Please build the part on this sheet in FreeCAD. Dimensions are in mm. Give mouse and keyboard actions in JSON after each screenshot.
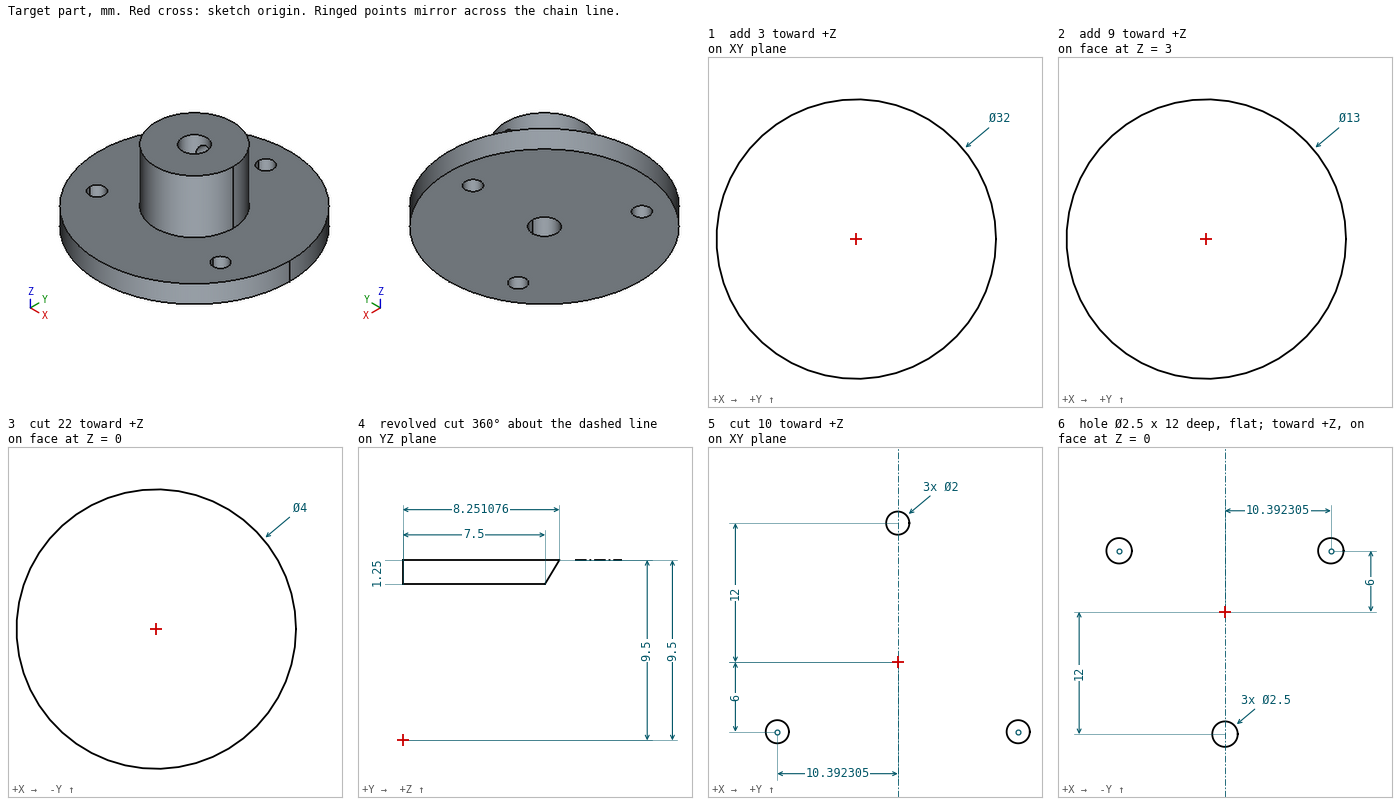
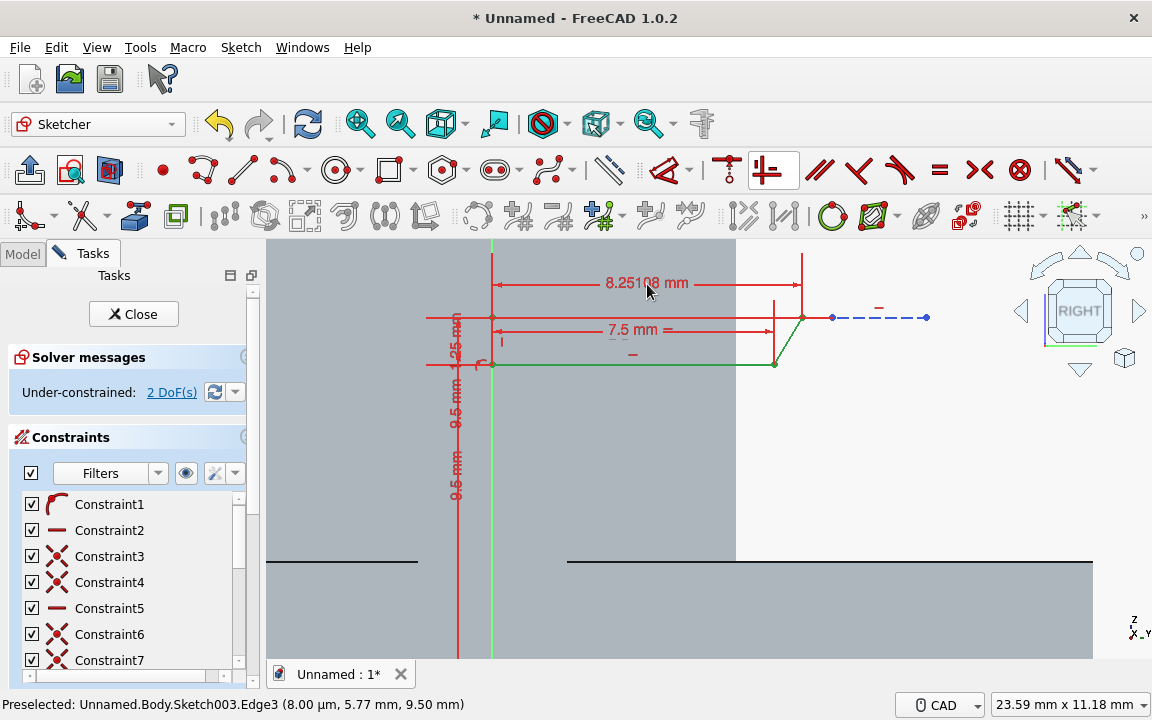
{"action": "left_click", "coordinate": [134, 314]}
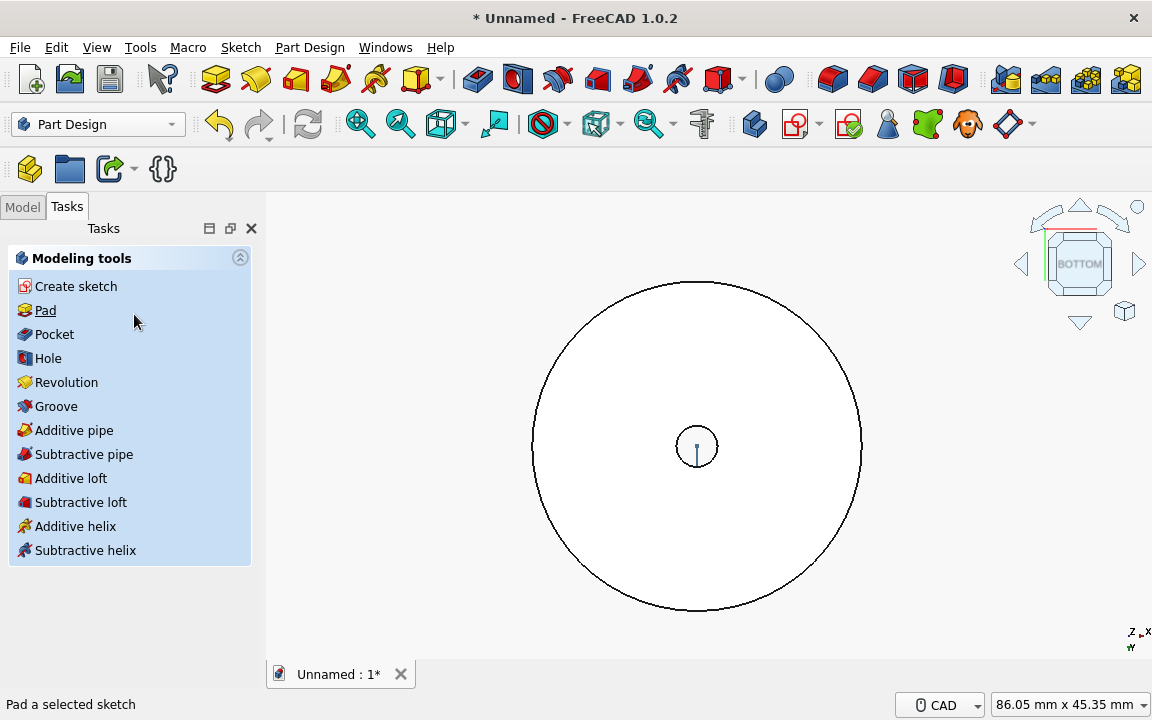
{"action": "left_click", "coordinate": [558, 80]}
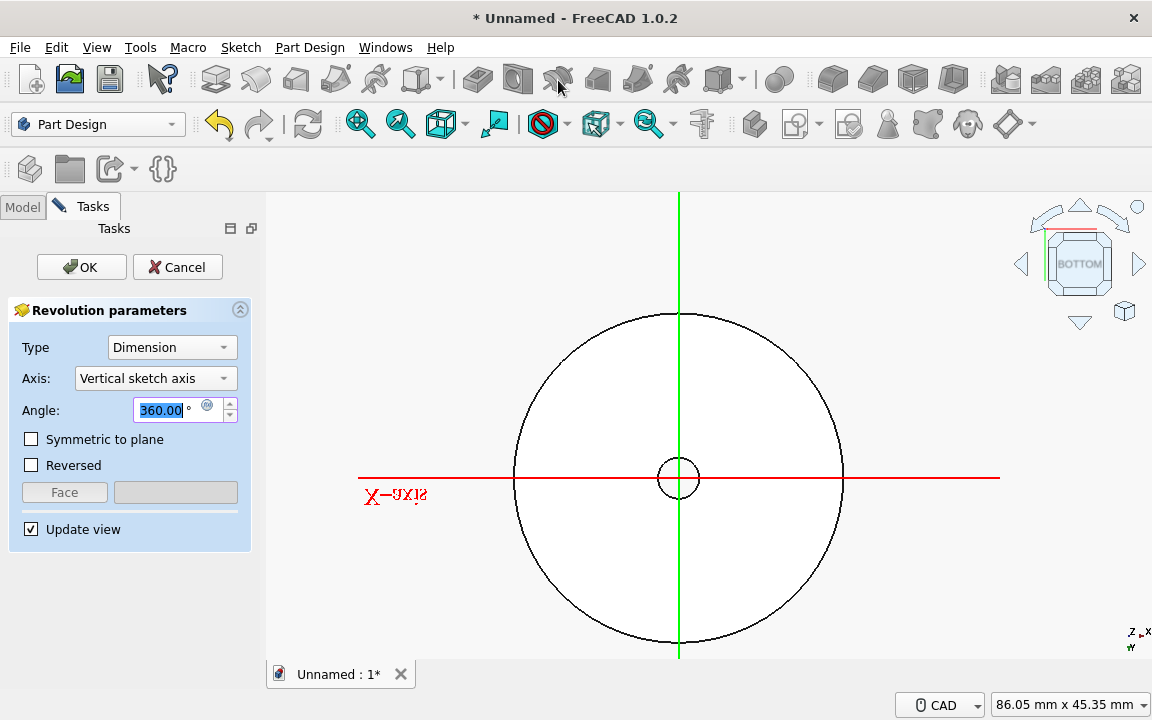
{"action": "left_click", "coordinate": [156, 378]}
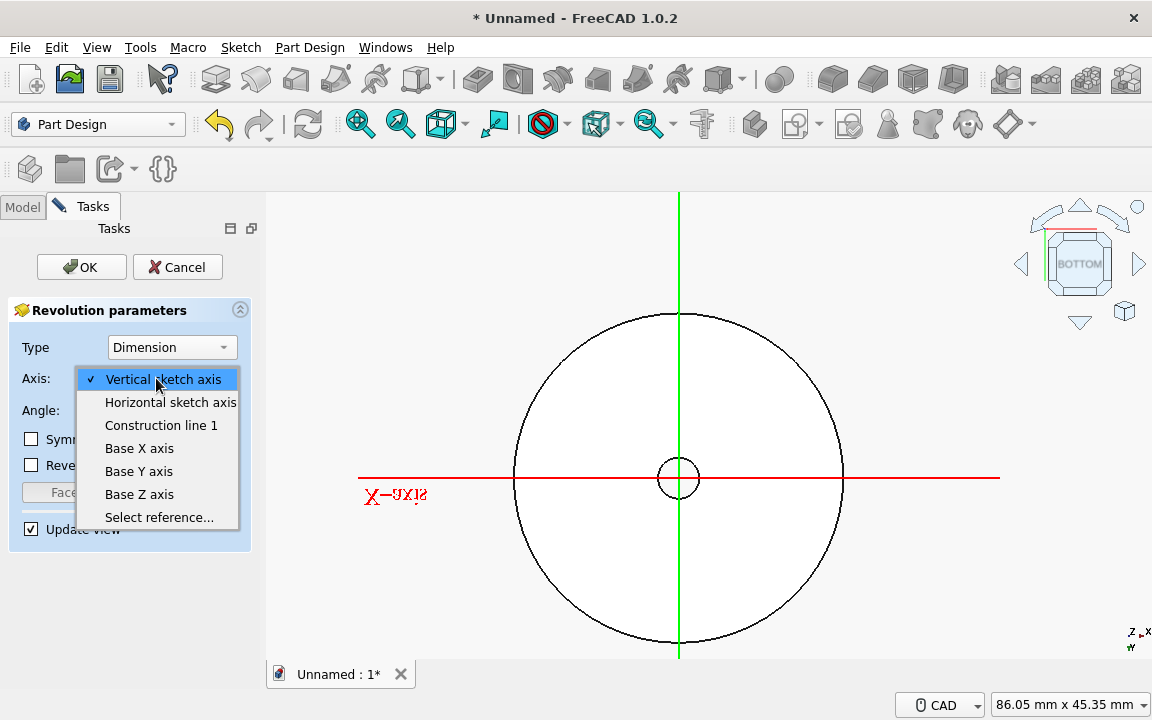
{"action": "left_click", "coordinate": [156, 426]}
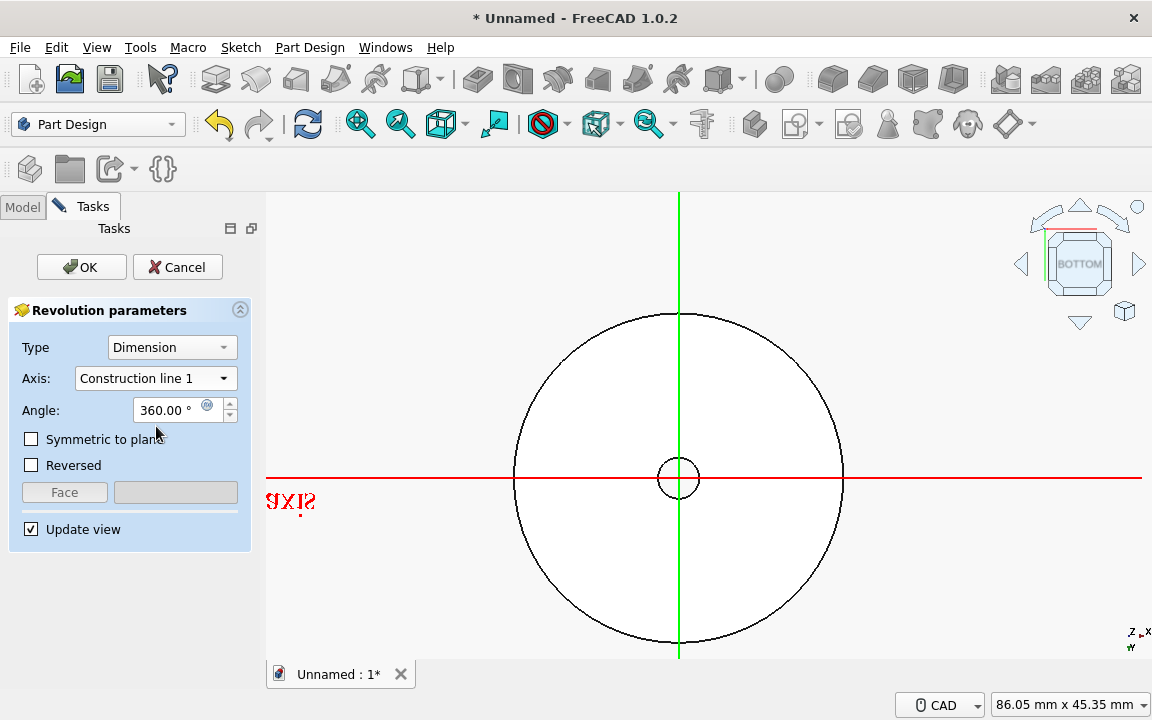
{"action": "left_click", "coordinate": [82, 267]}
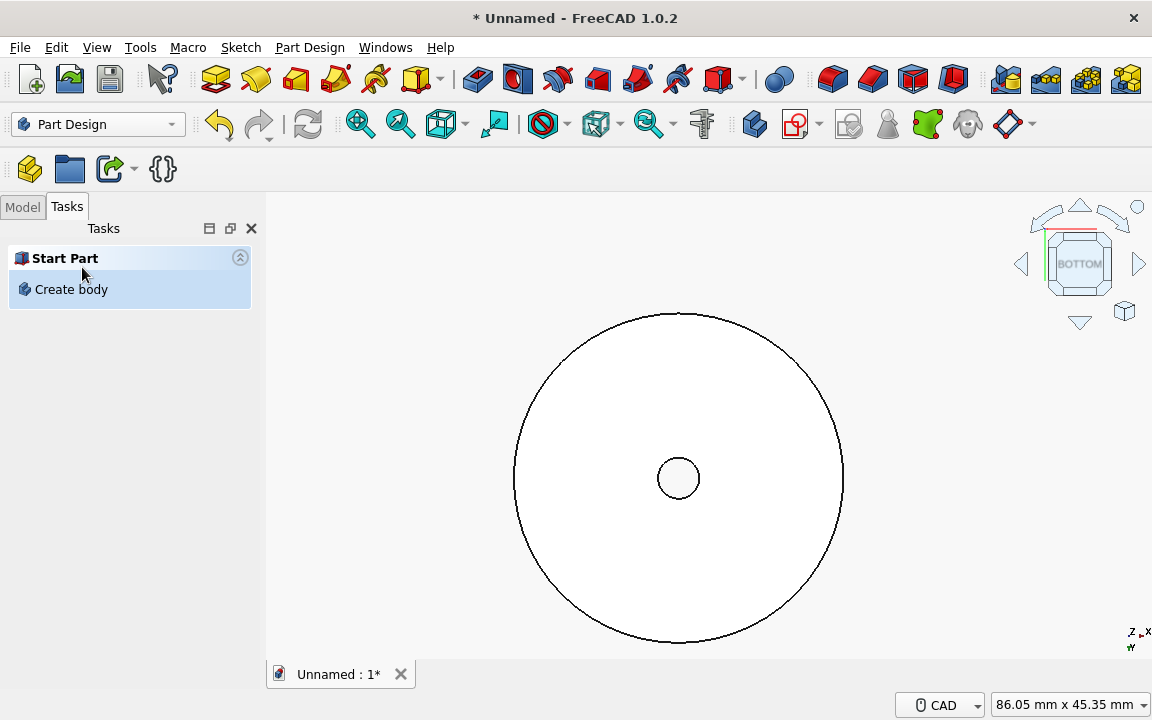
{"action": "left_click", "coordinate": [796, 124]}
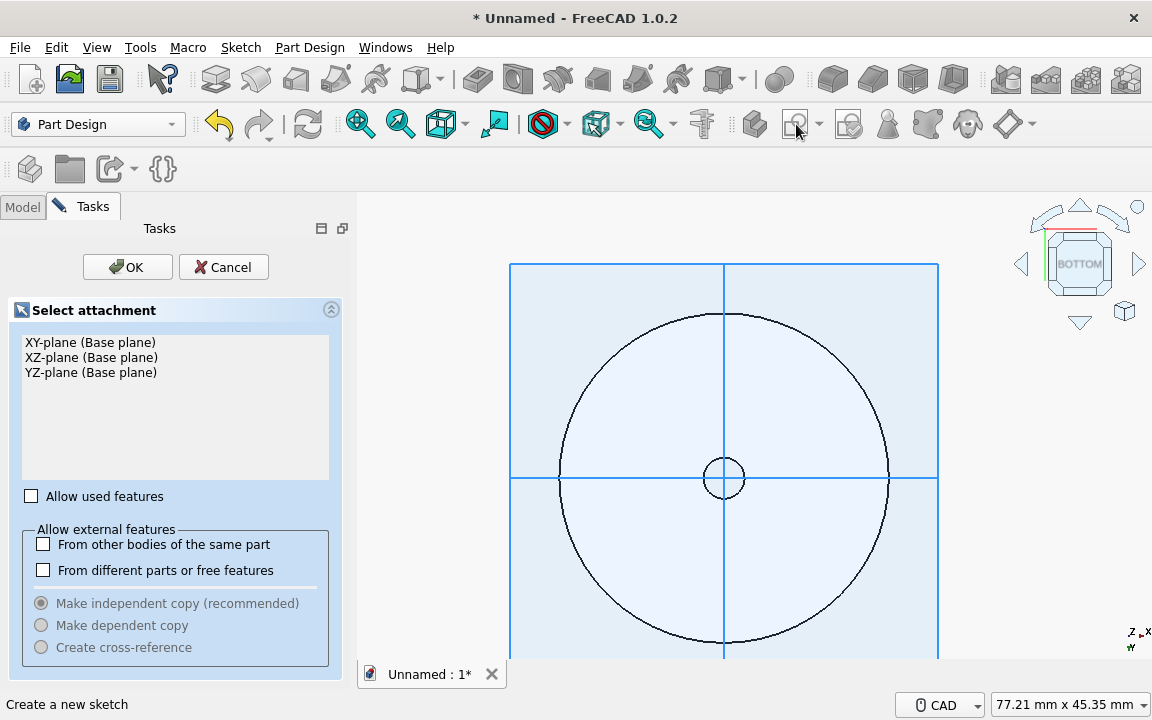
{"action": "left_click", "coordinate": [82, 342]}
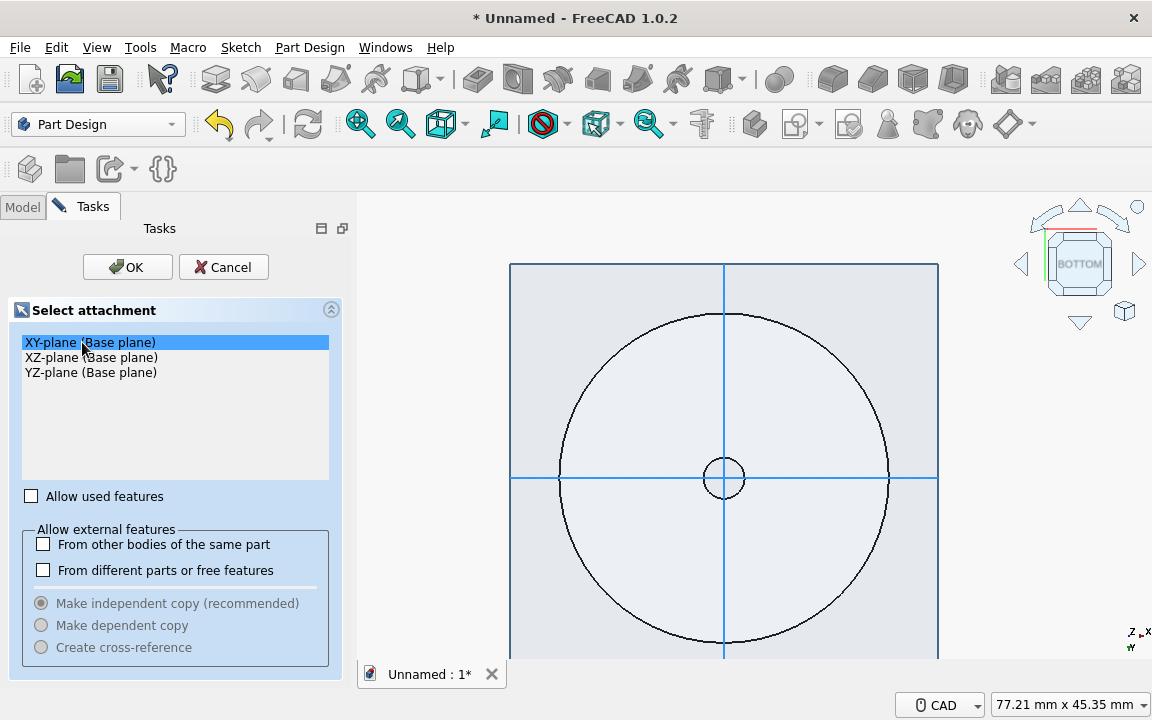
{"action": "left_click", "coordinate": [128, 267]}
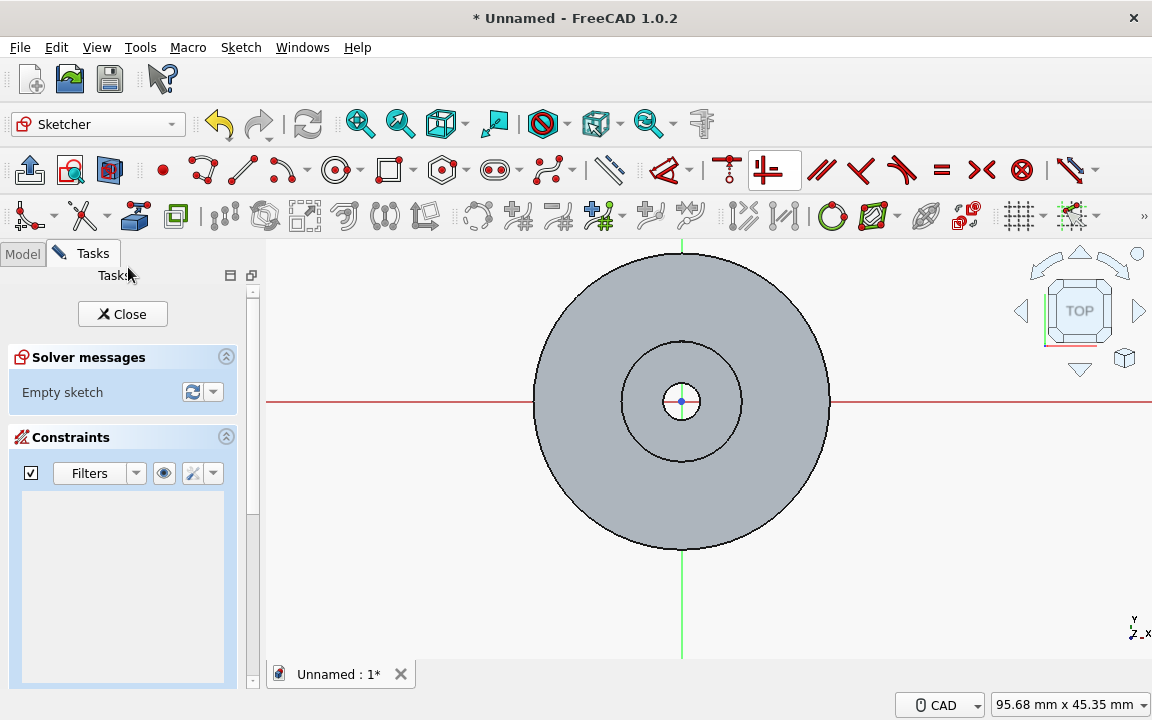
{"action": "left_click", "coordinate": [110, 170]}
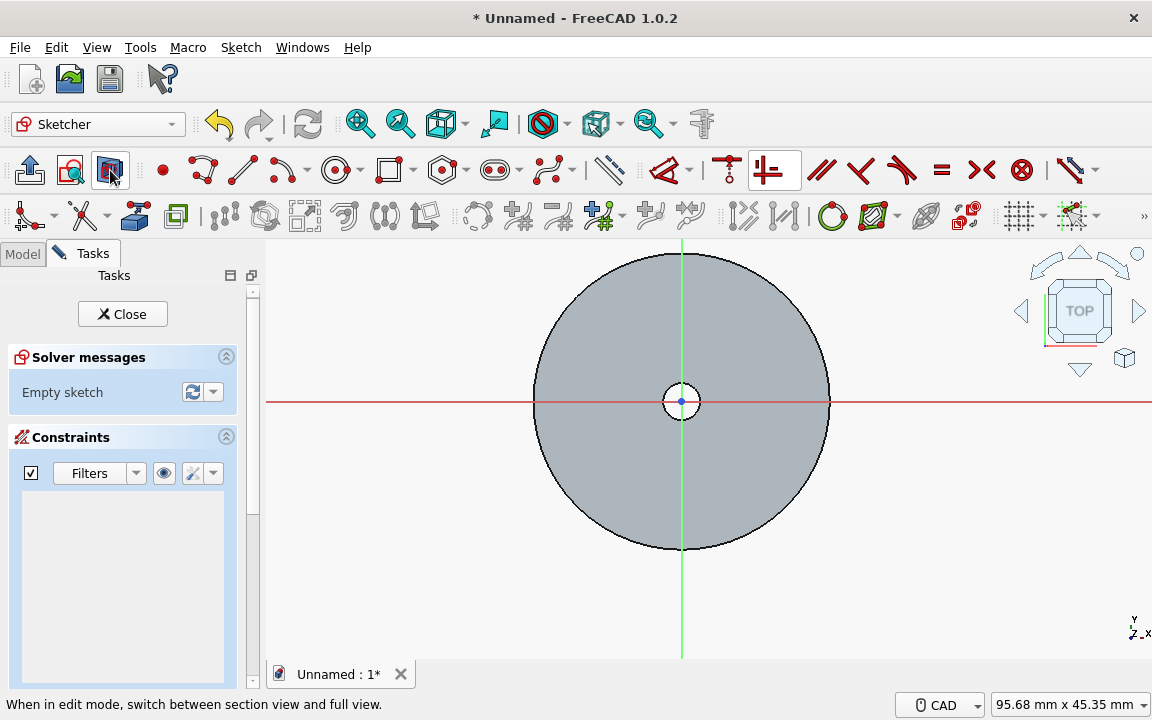
{"action": "scroll", "coordinate": [455, 631], "scroll_direction": "down", "scroll_amount": 1}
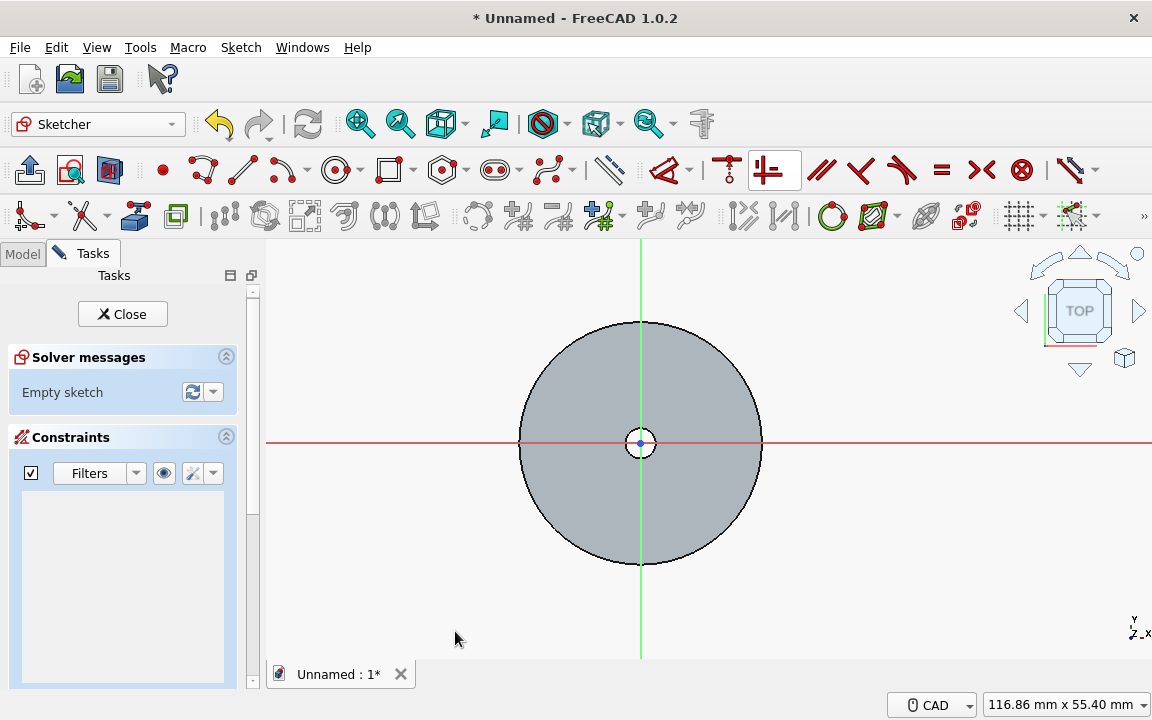
{"action": "scroll", "coordinate": [641, 386], "scroll_direction": "up", "scroll_amount": 3}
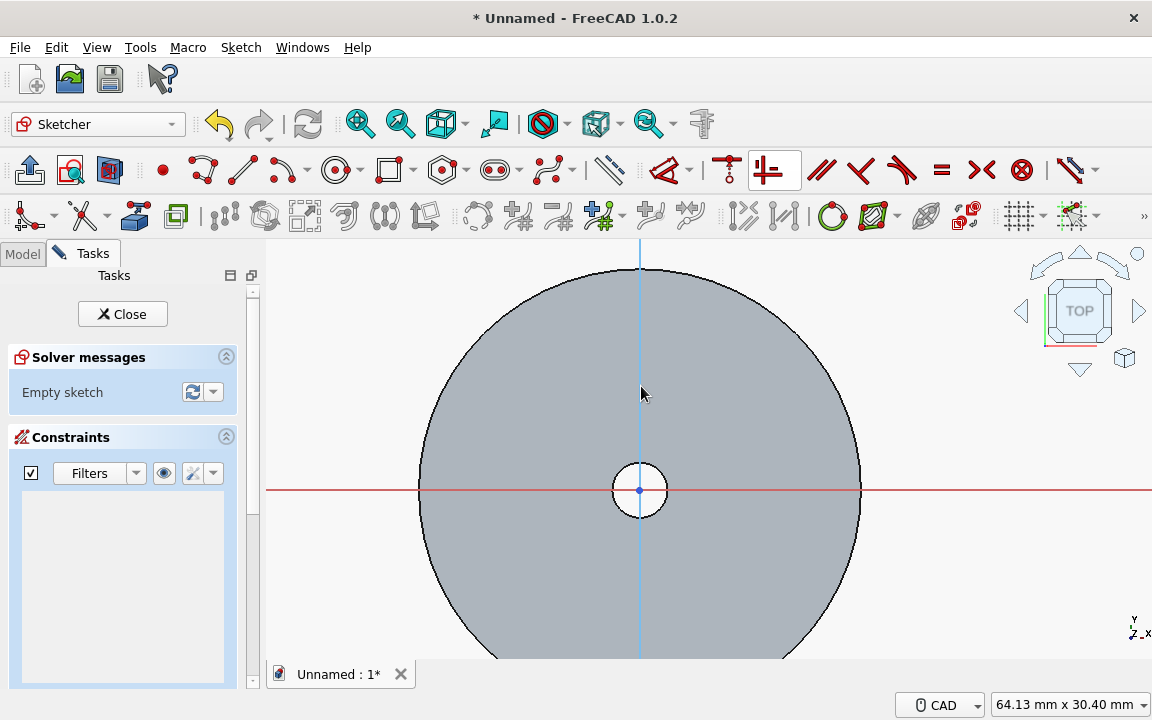
{"action": "left_click", "coordinate": [336, 170]}